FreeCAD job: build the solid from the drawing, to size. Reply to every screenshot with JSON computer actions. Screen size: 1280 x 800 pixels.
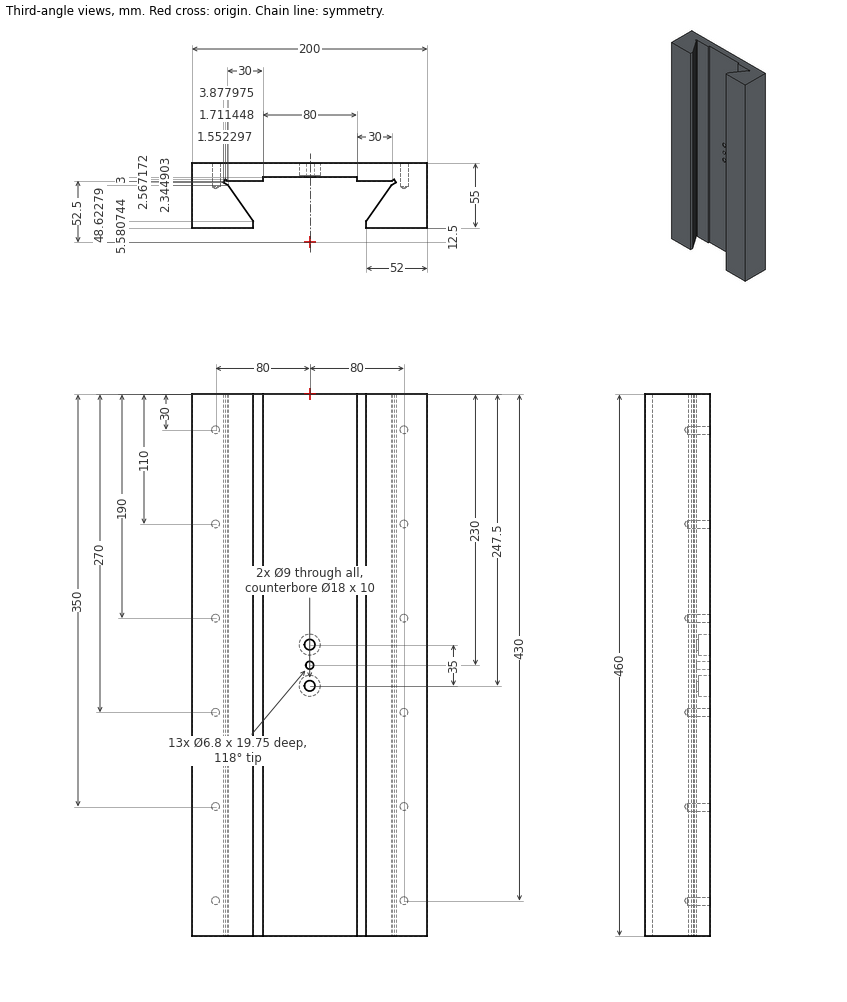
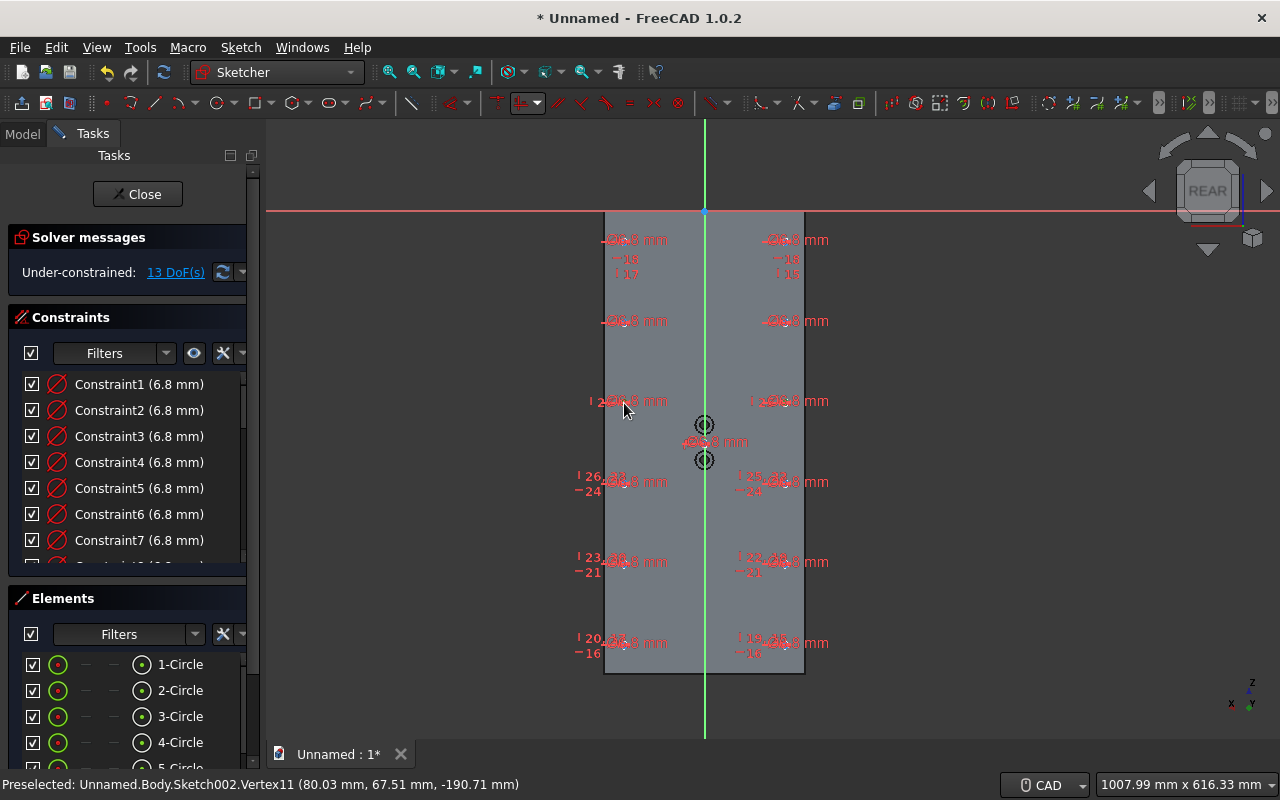
{"action": "left_click", "coordinate": [540, 104]}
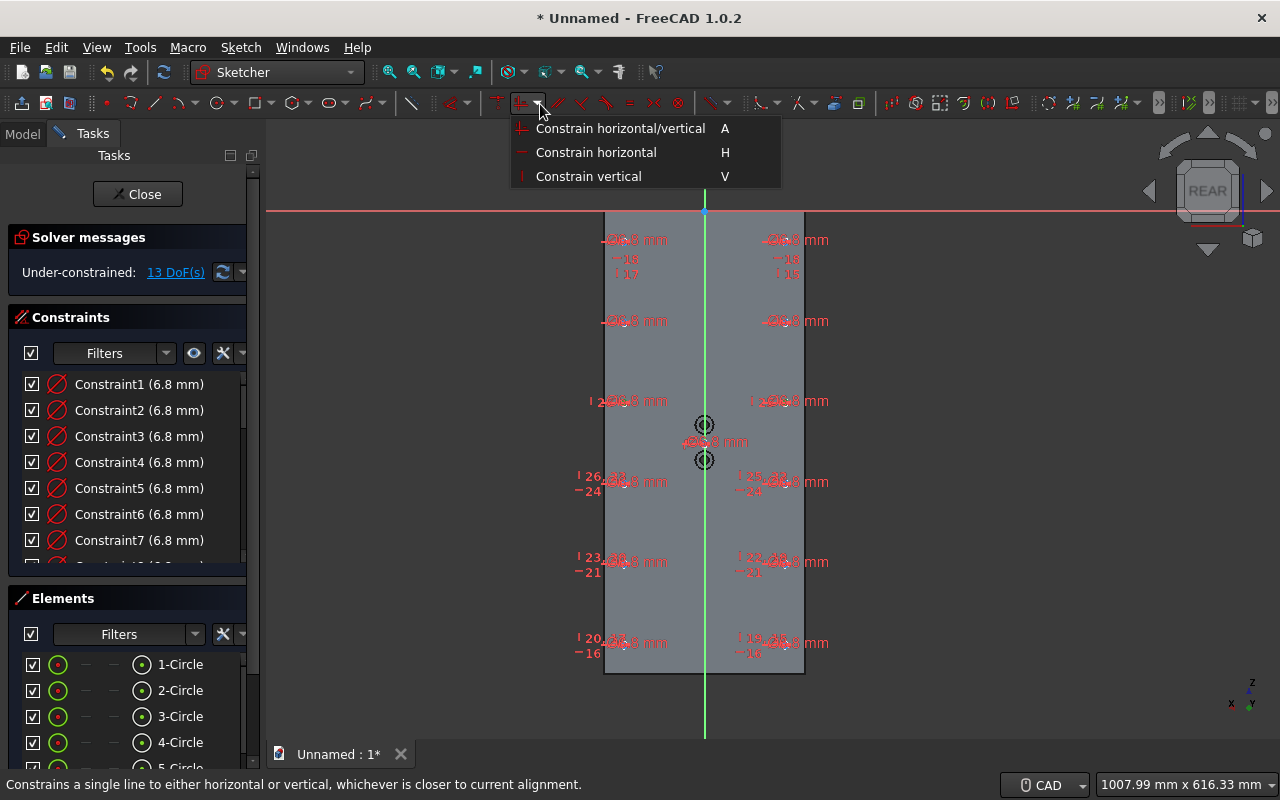
{"action": "left_click", "coordinate": [646, 152]}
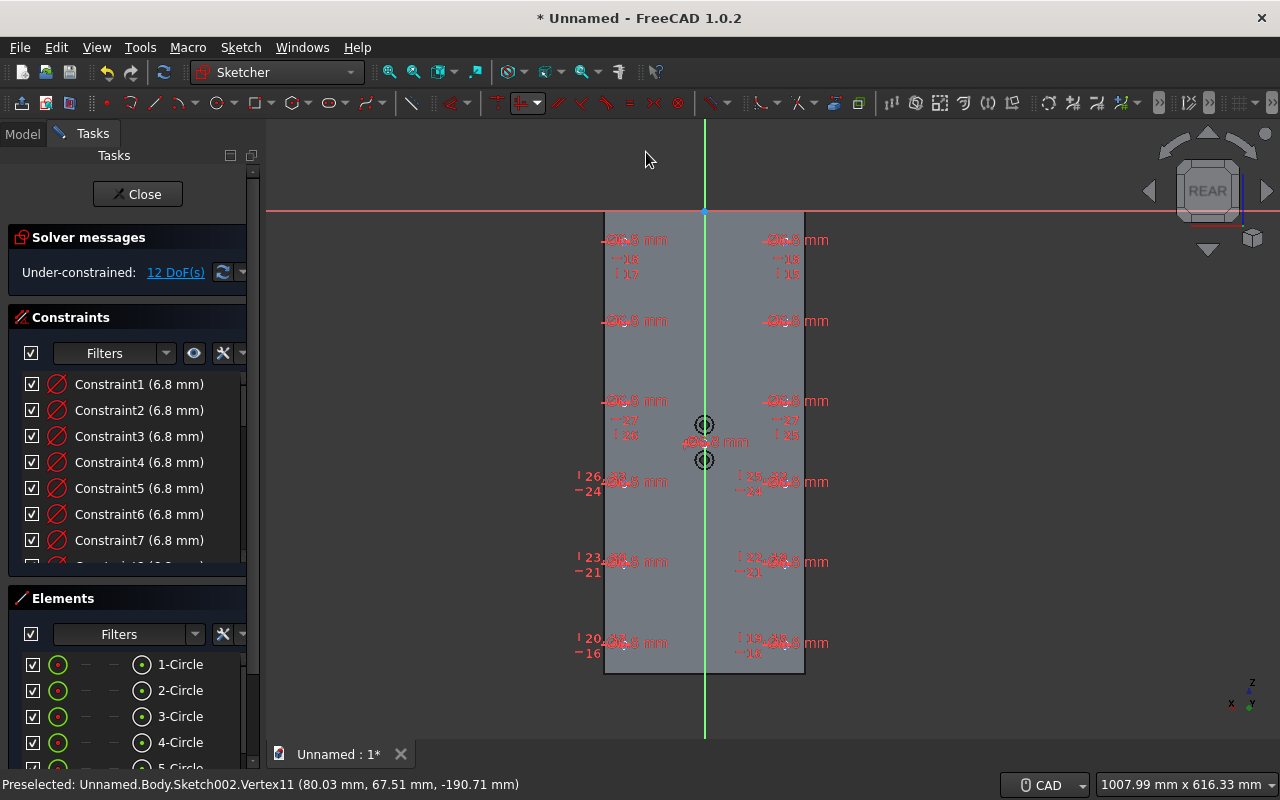
{"action": "left_click", "coordinate": [785, 242]}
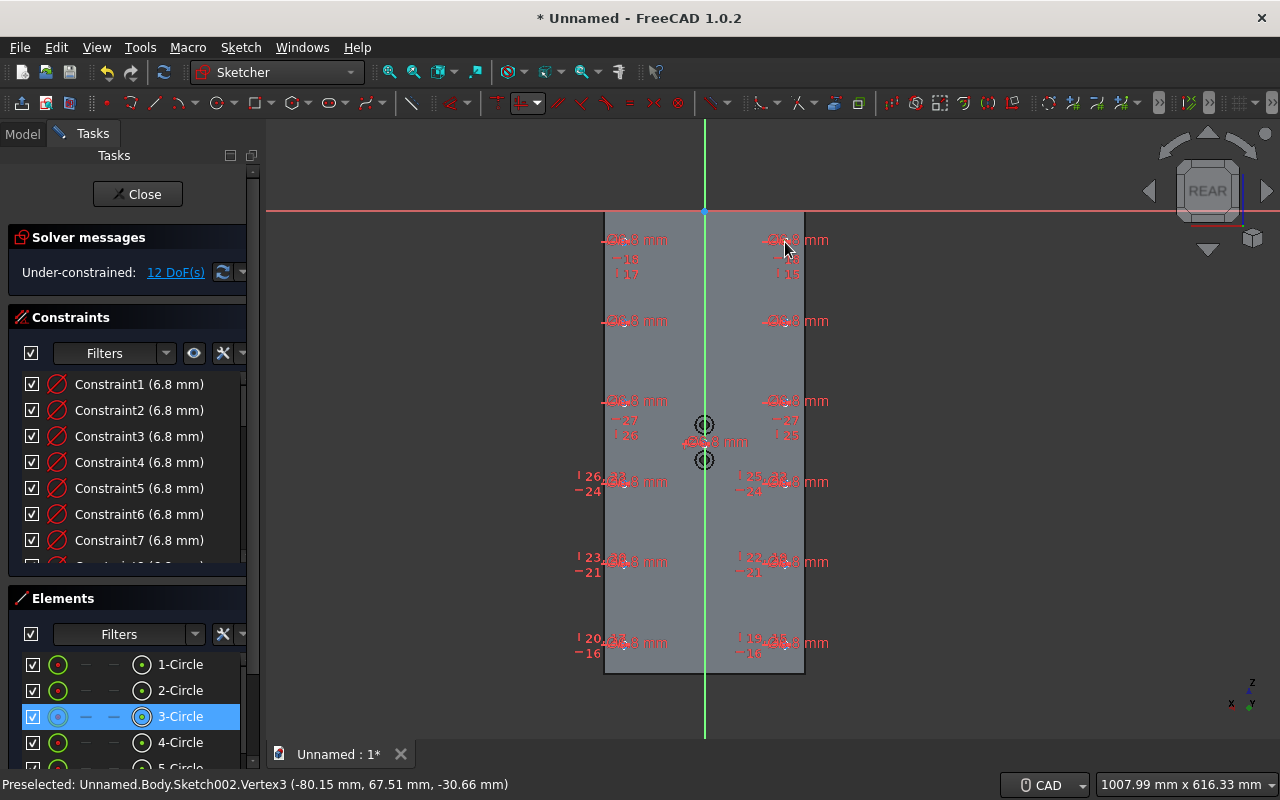
{"action": "left_click", "coordinate": [785, 323]}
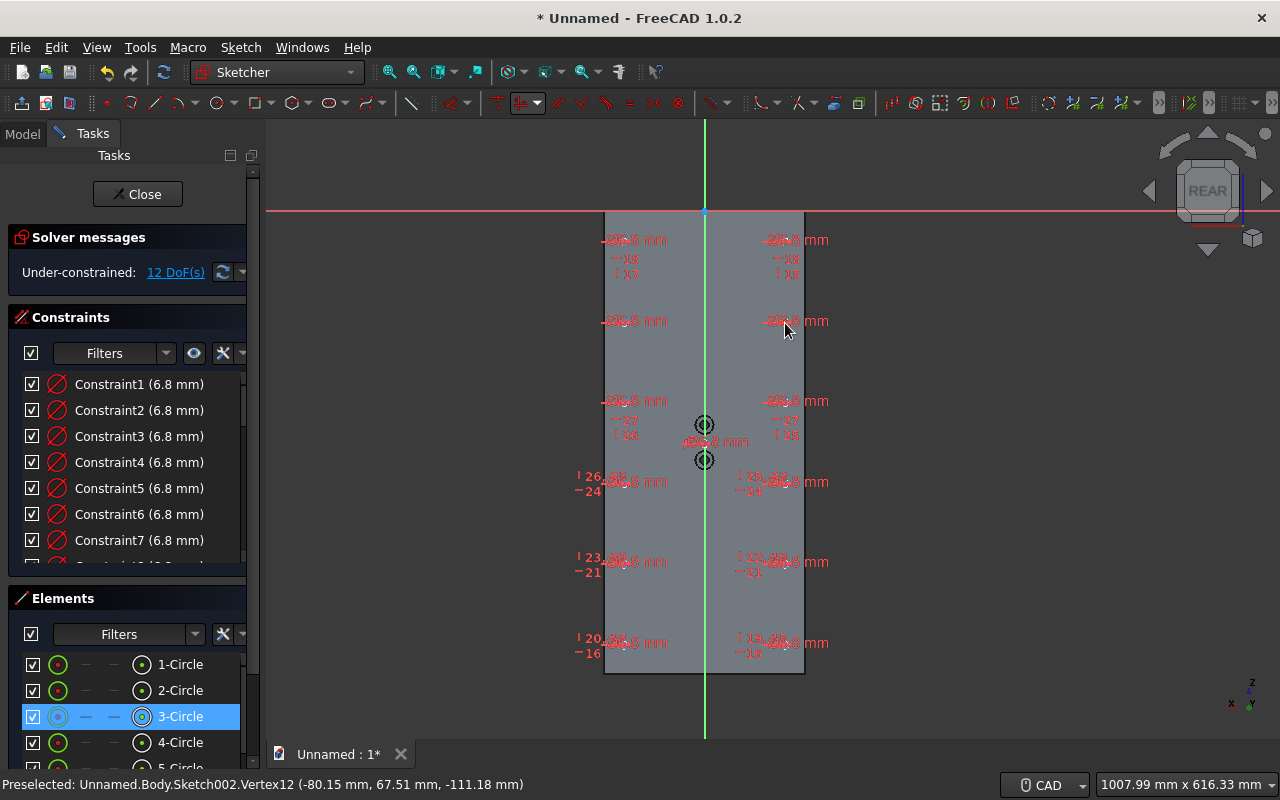
{"action": "key", "text": "v"}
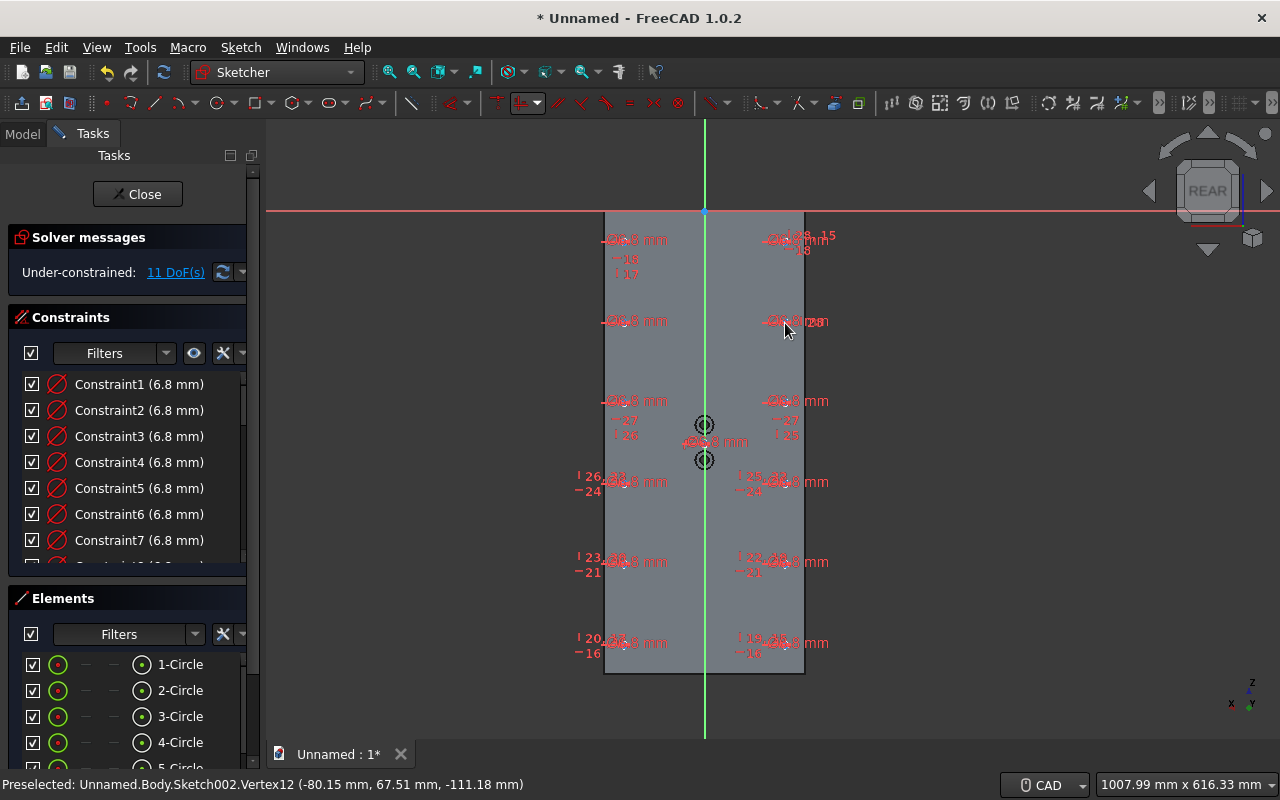
{"action": "left_click", "coordinate": [624, 242]}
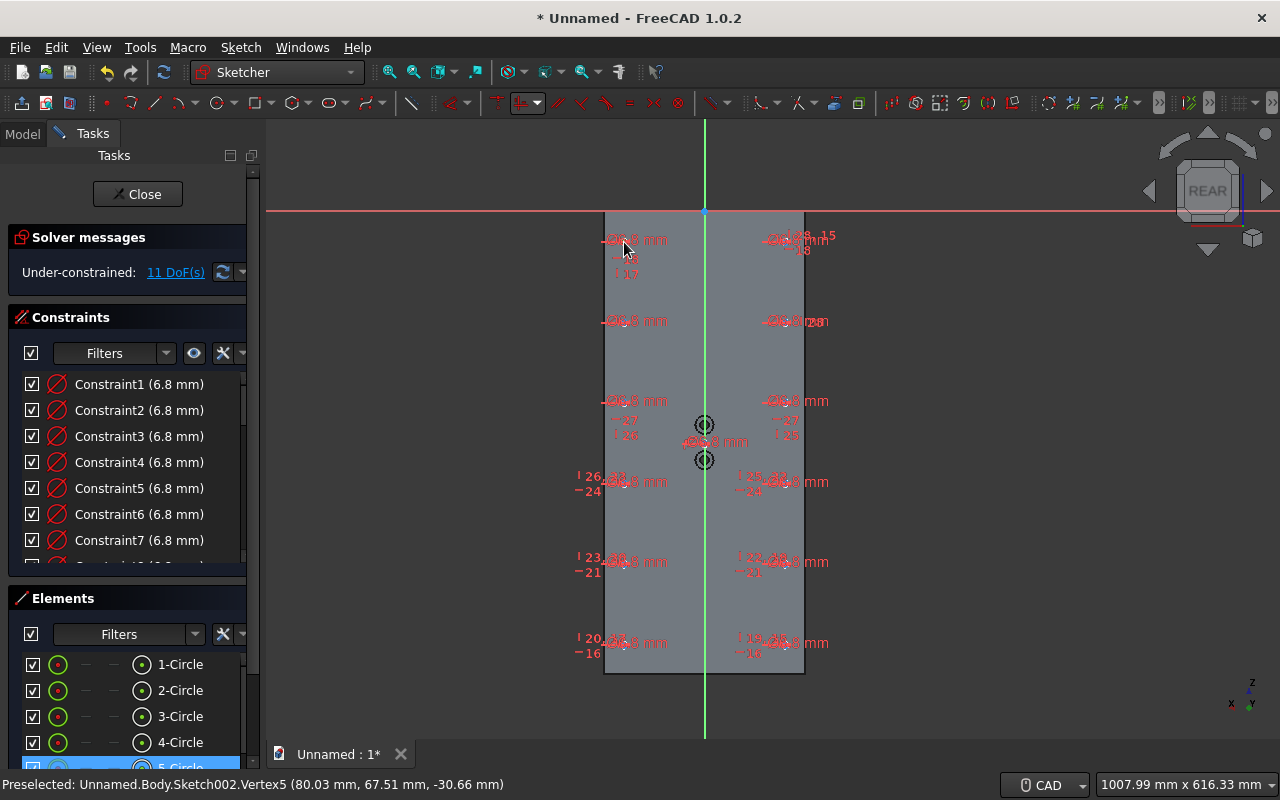
{"action": "left_click", "coordinate": [624, 323]}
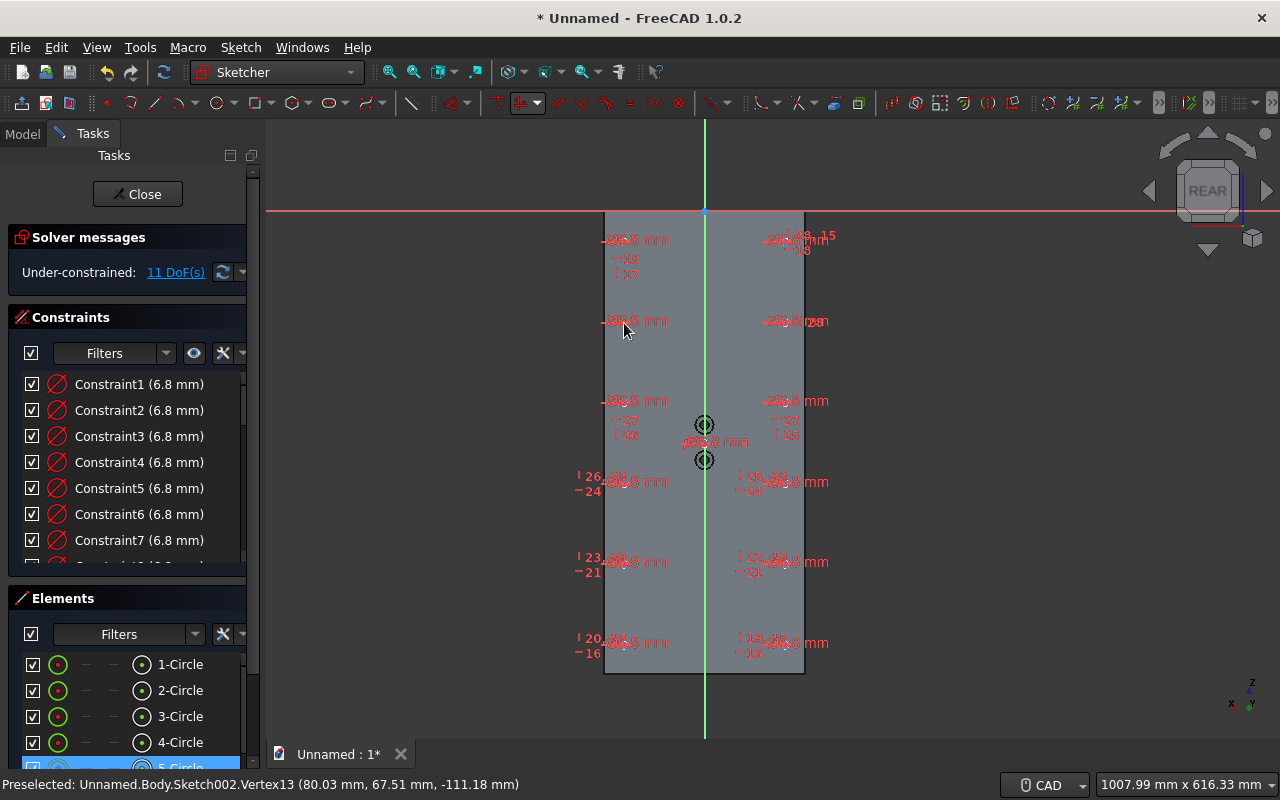
{"action": "key", "text": "v"}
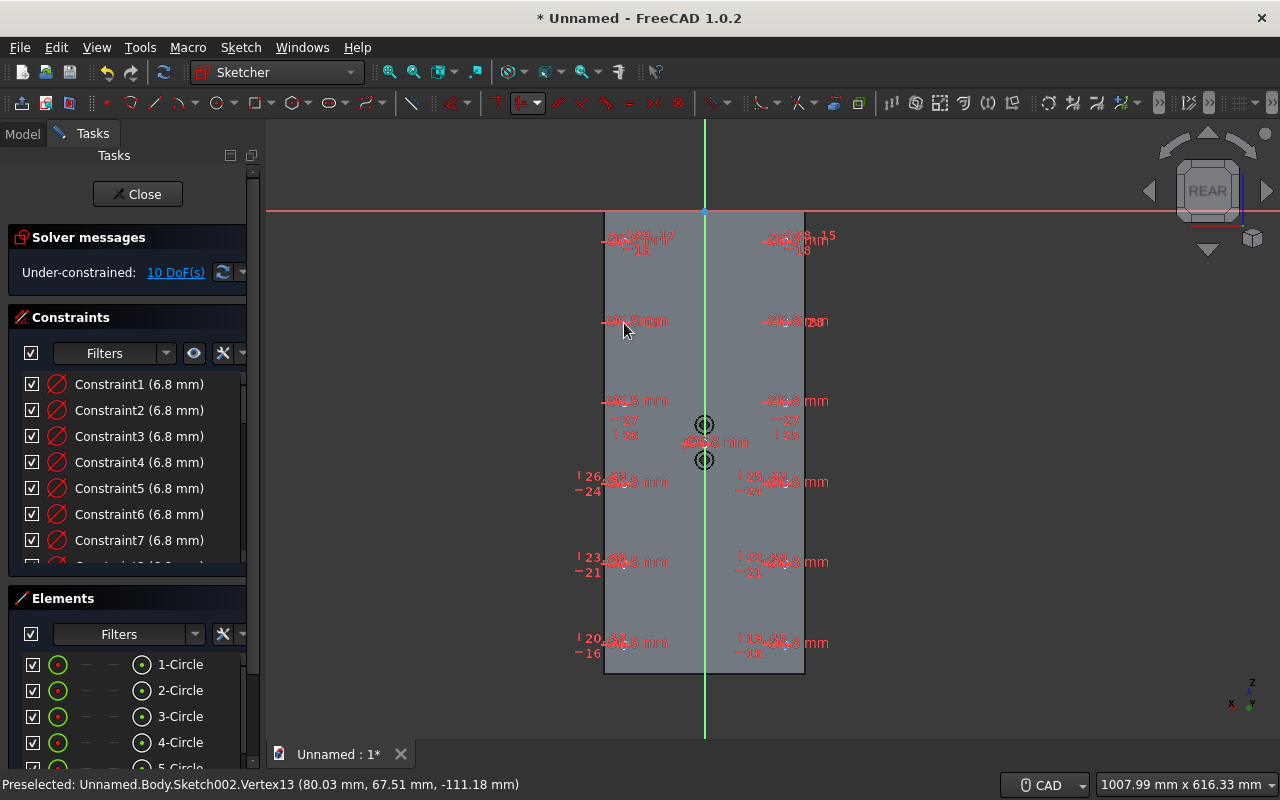
{"action": "left_click", "coordinate": [785, 323]}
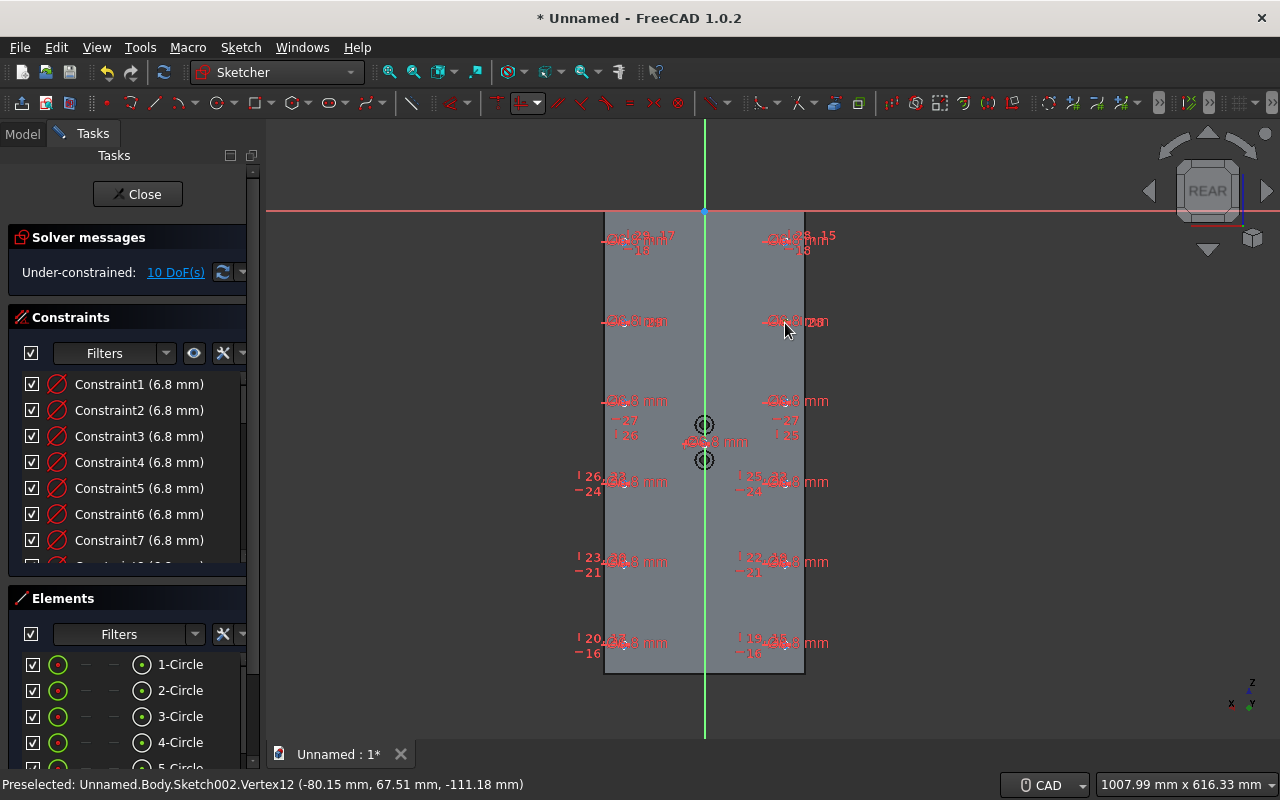
{"action": "left_click", "coordinate": [624, 323]}